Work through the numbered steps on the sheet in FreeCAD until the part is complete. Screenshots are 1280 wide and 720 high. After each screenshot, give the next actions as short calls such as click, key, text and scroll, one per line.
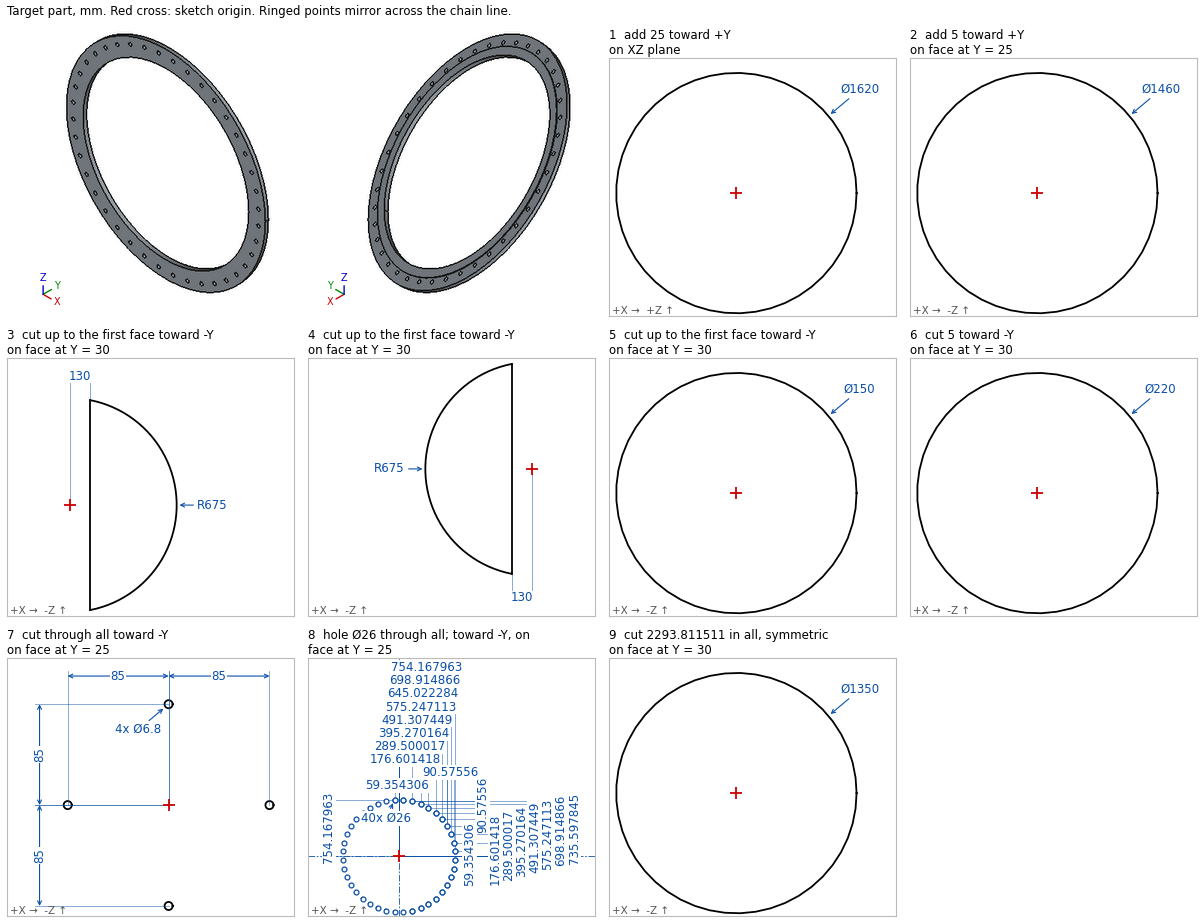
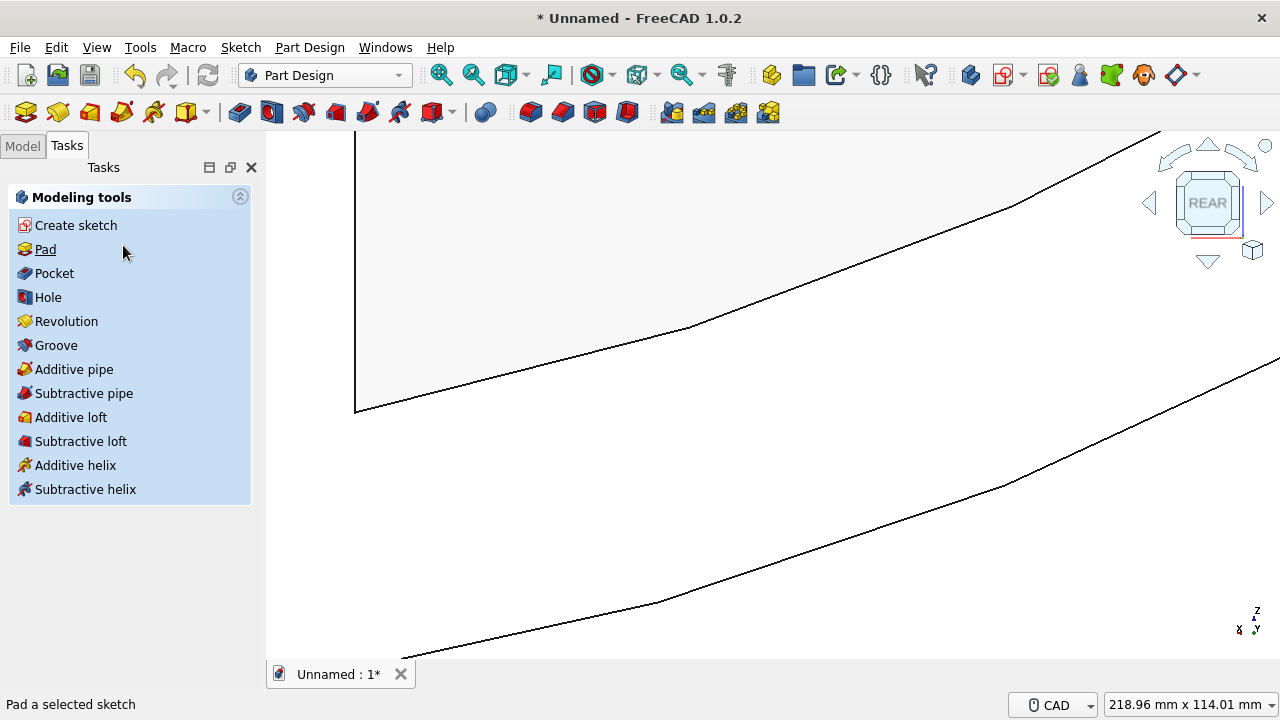
click(240, 112)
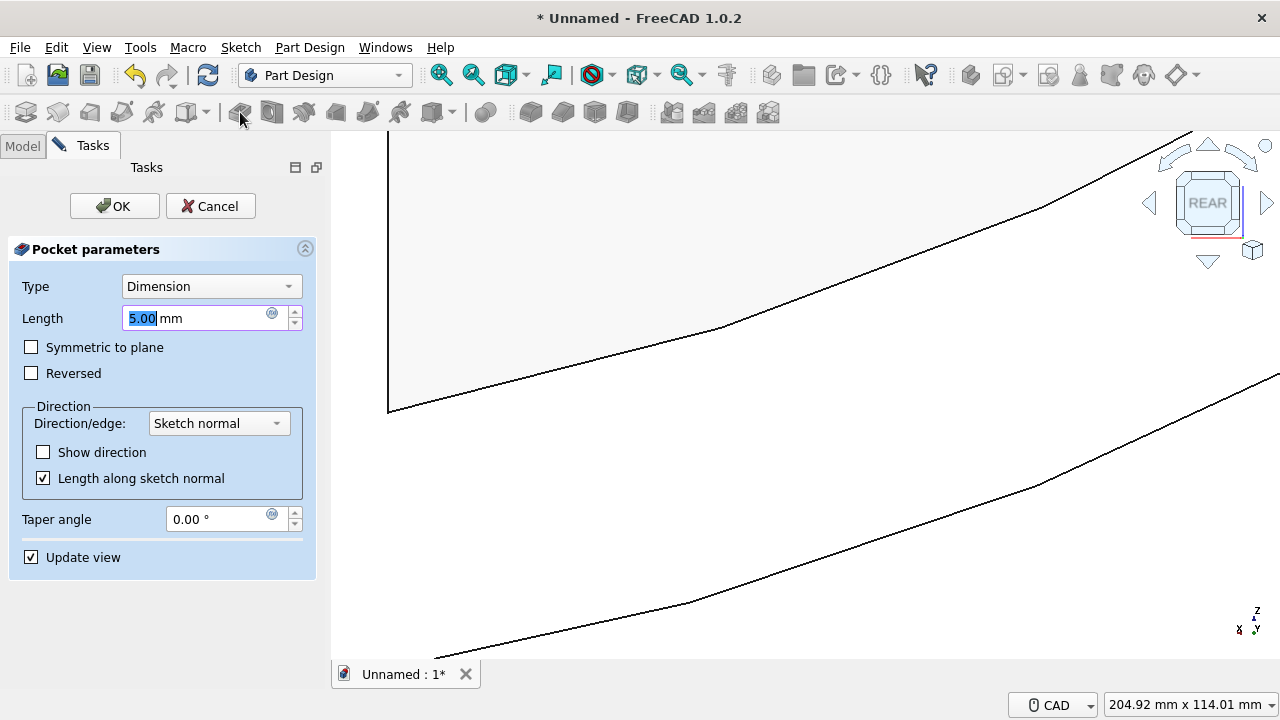
click(212, 286)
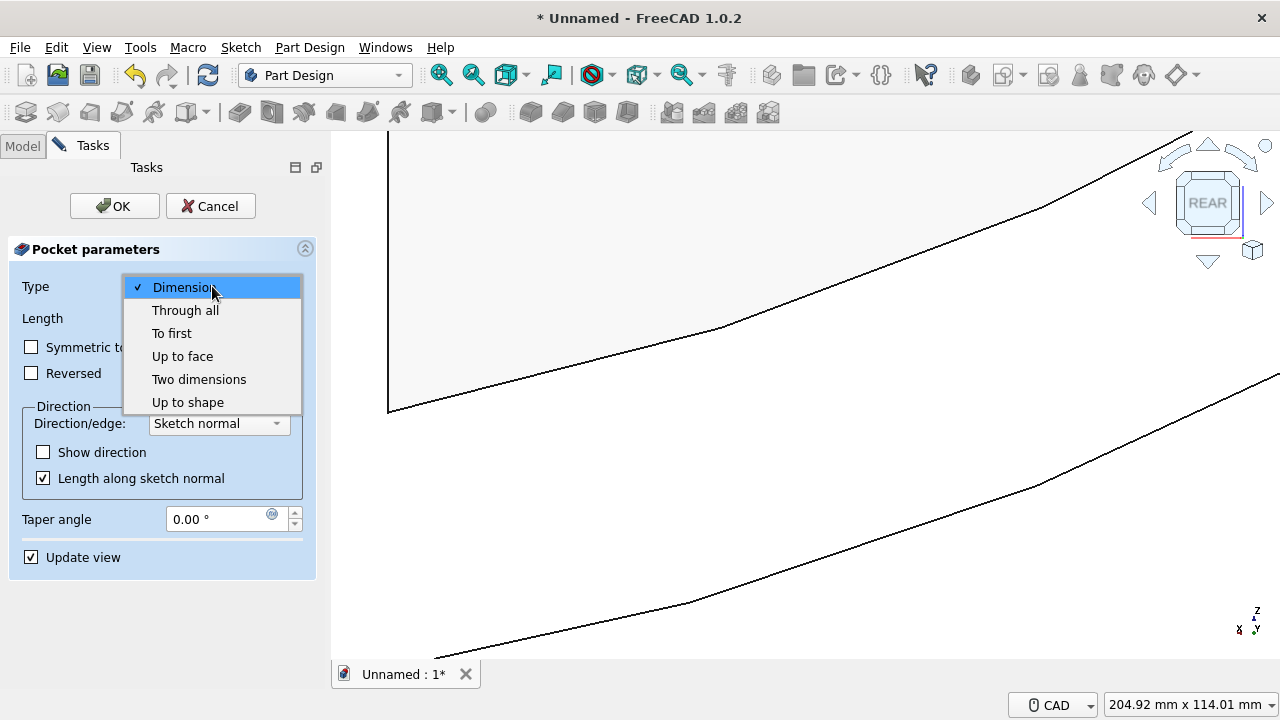
click(212, 310)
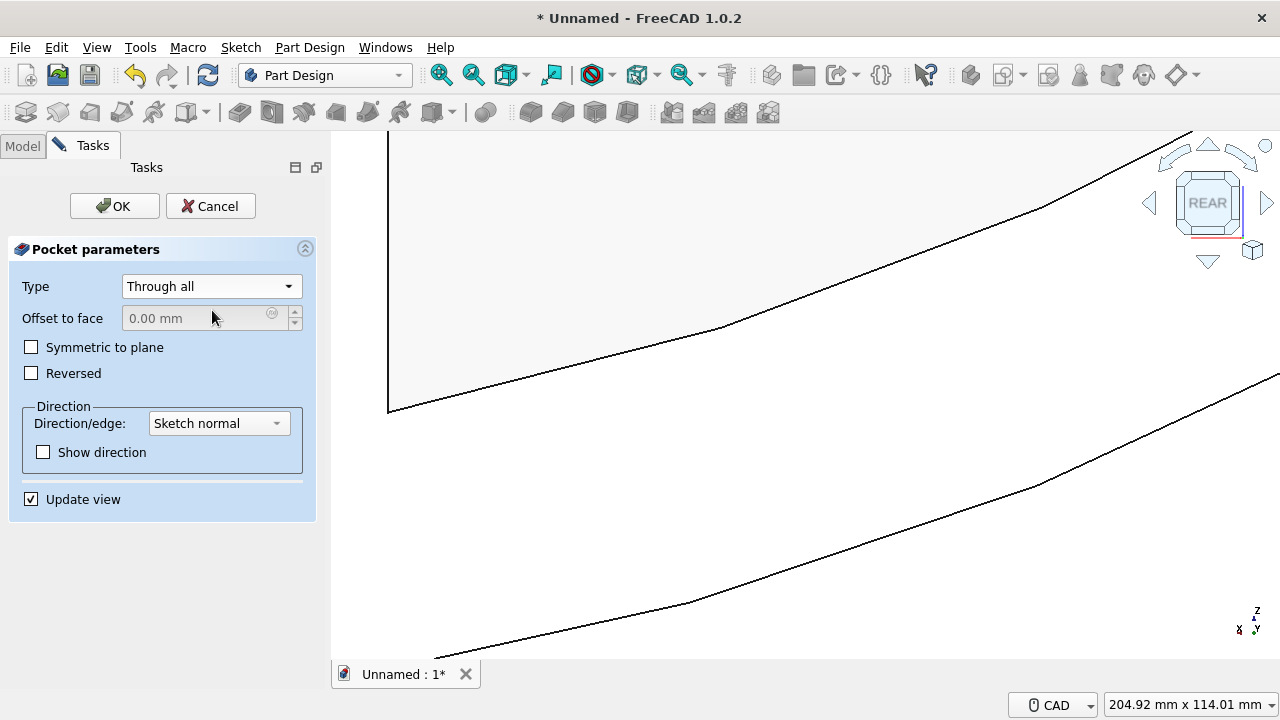
click(115, 206)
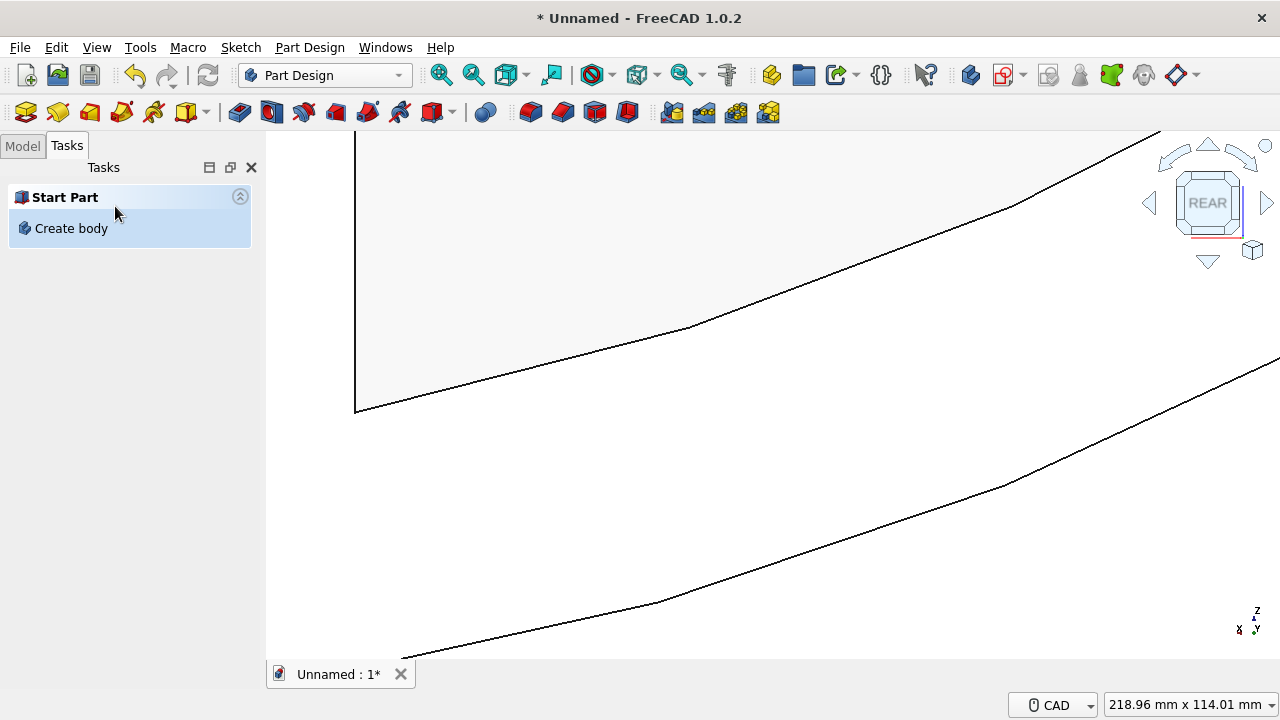
click(442, 76)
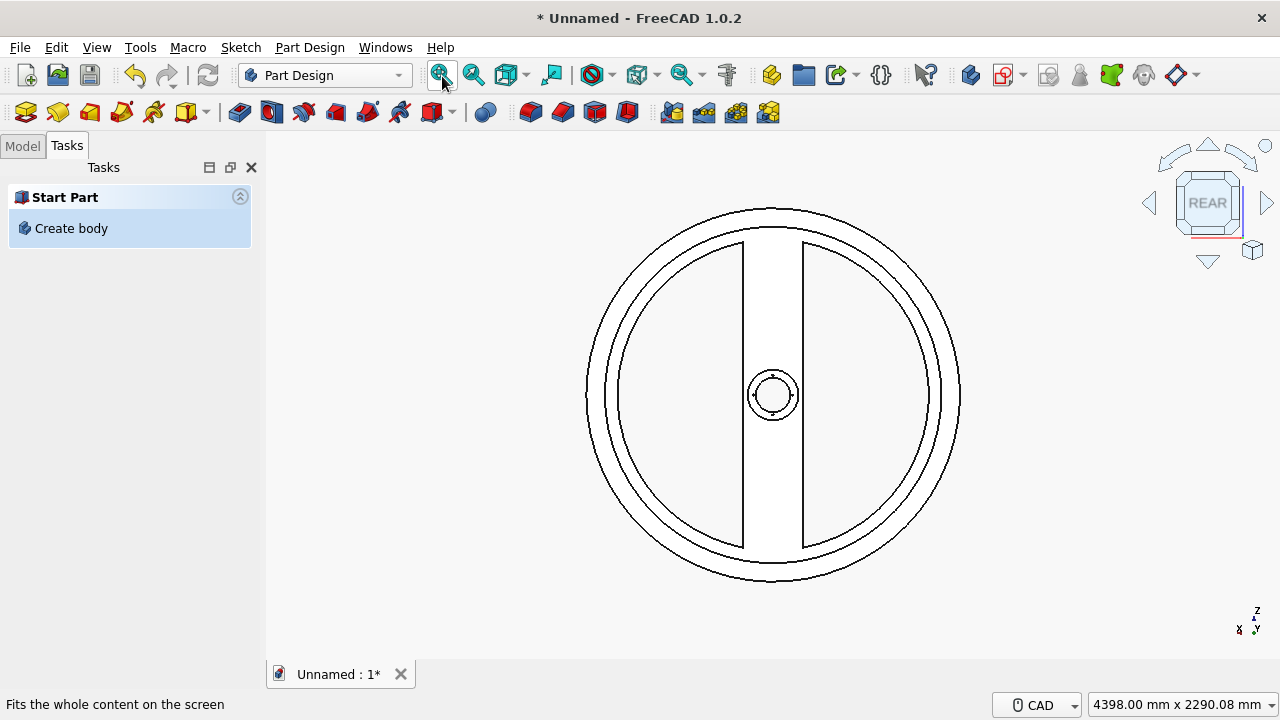
scroll(826, 554, up, 15)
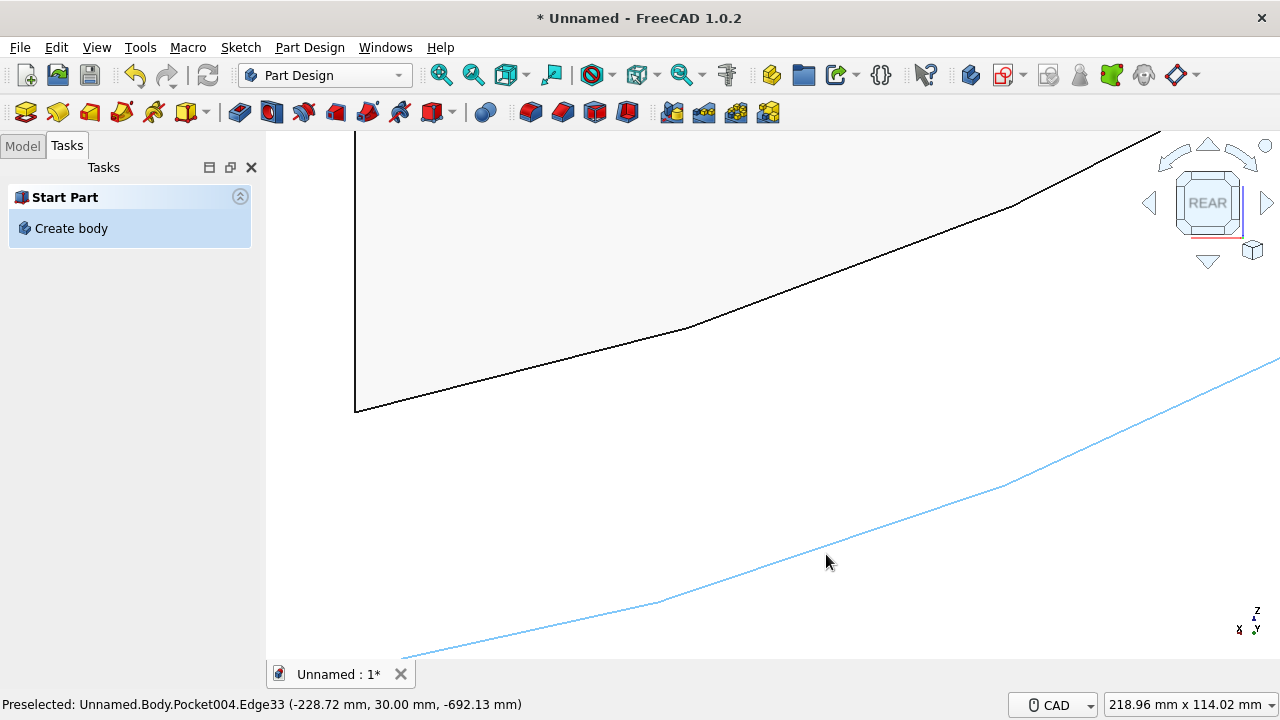
click(825, 559)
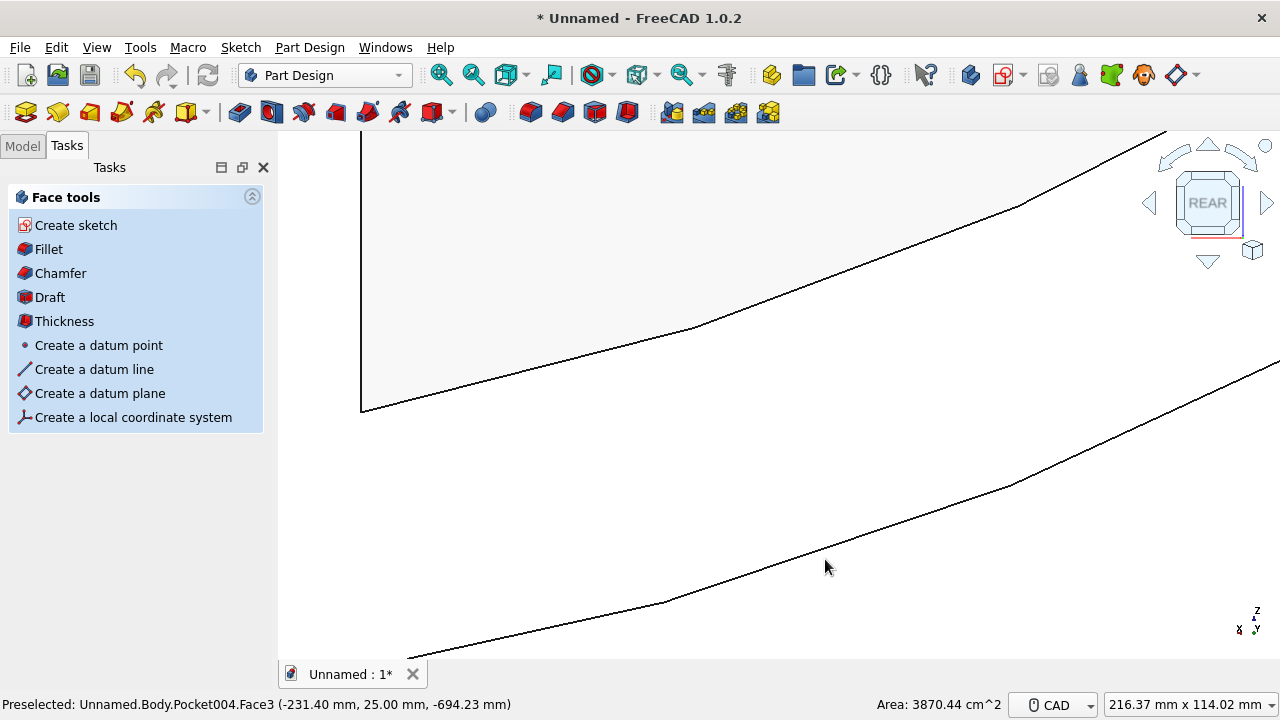
click(1004, 76)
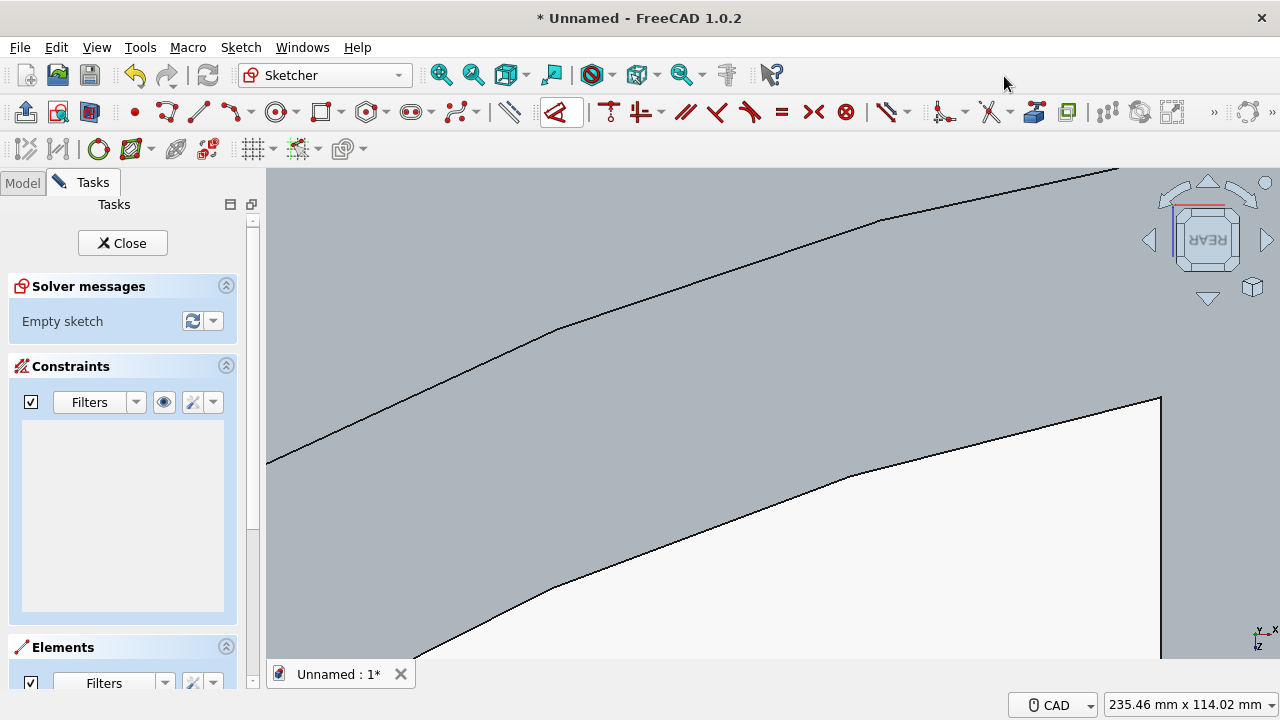
scroll(651, 265, down, 15)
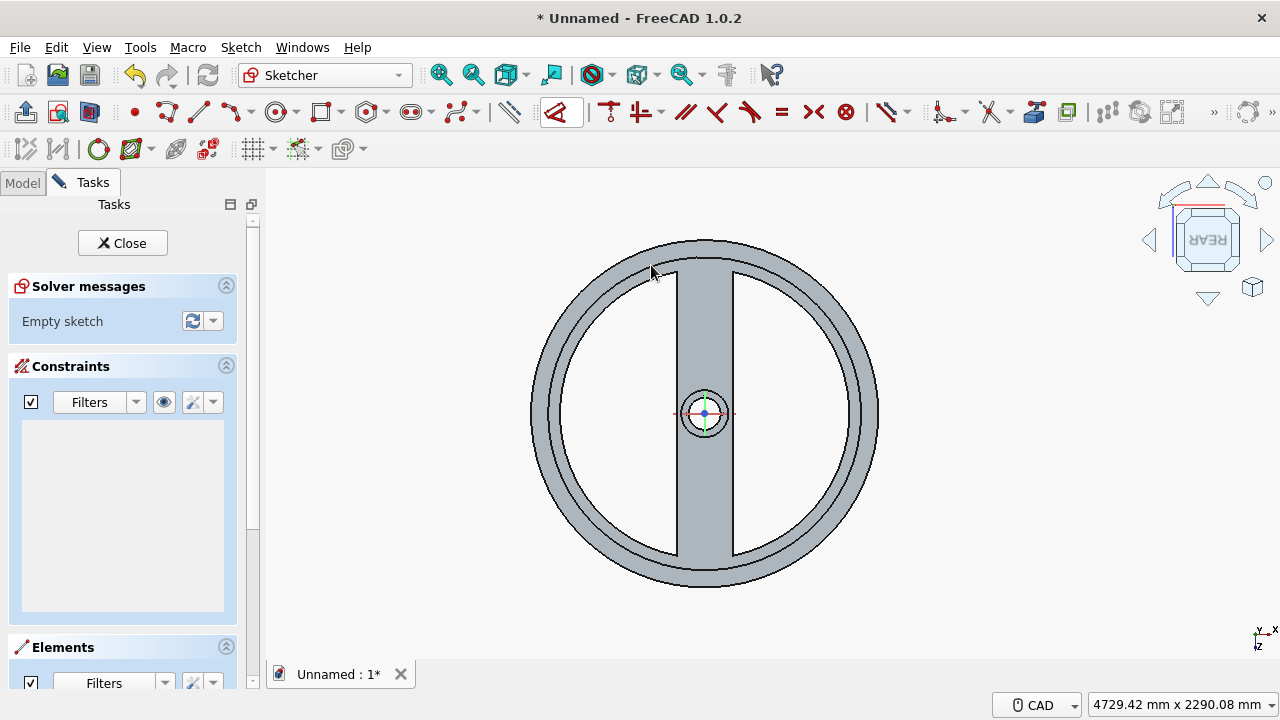
click(276, 112)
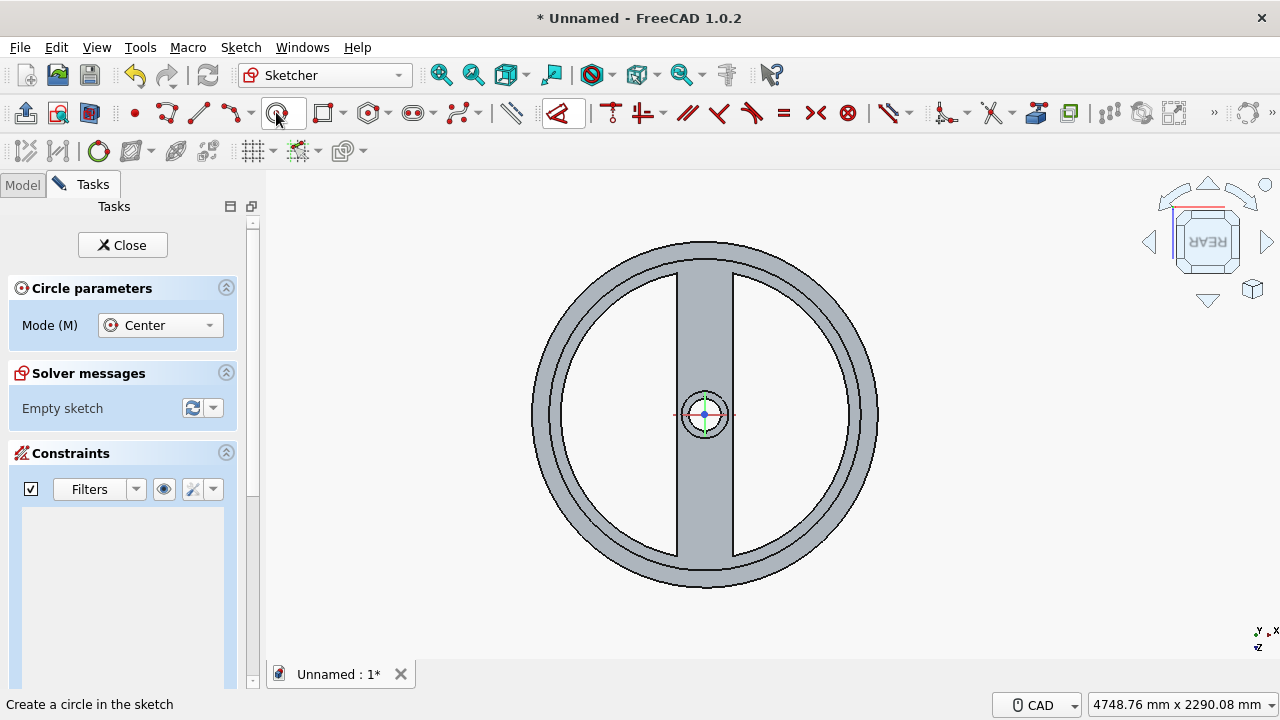
scroll(692, 254, up, 11)